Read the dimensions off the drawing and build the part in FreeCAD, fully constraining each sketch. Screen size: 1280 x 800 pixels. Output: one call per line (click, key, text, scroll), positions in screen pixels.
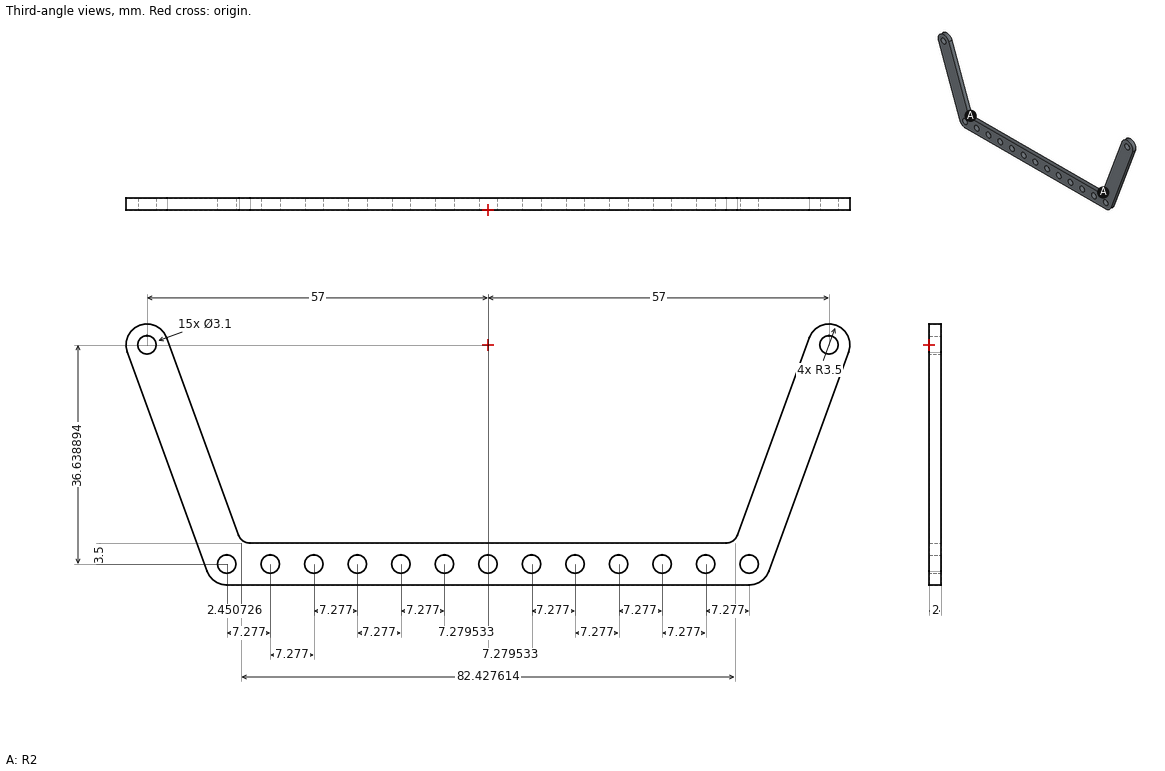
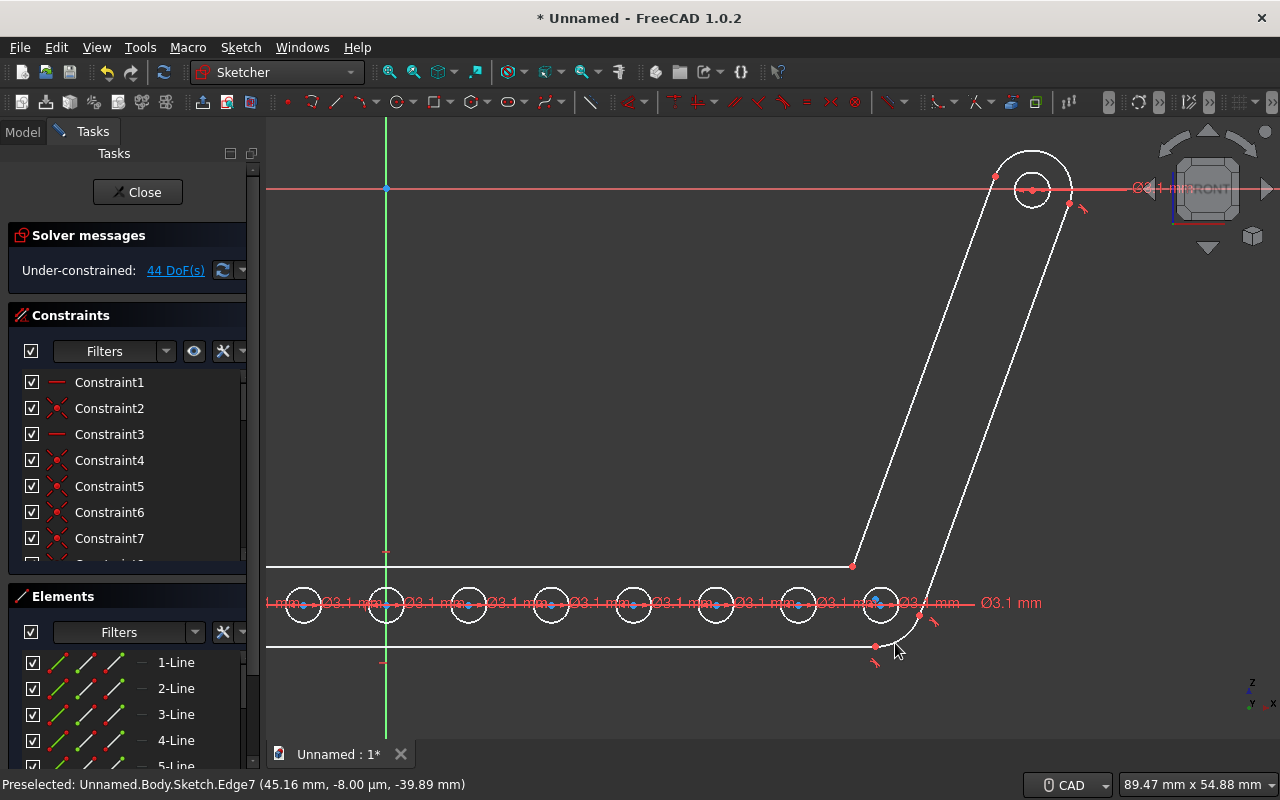
click(580, 647)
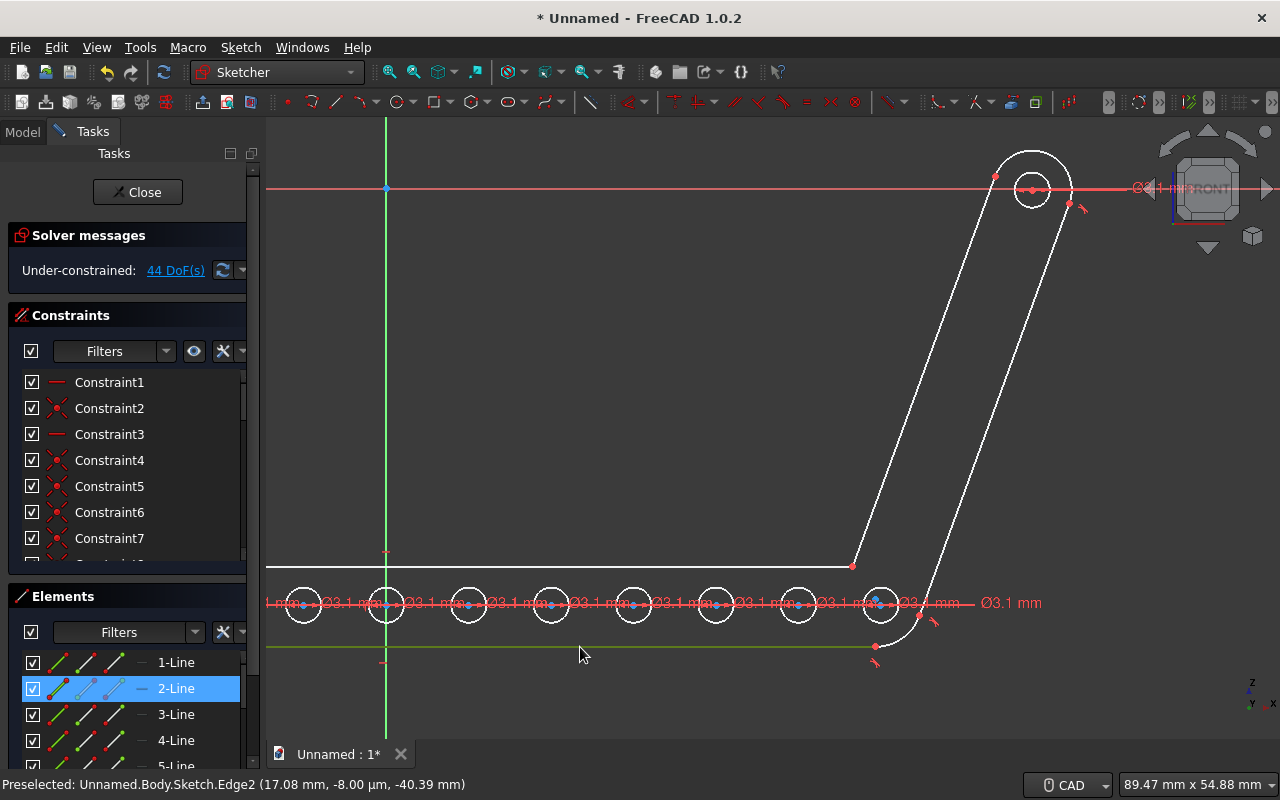
scroll(964, 453, down, 4)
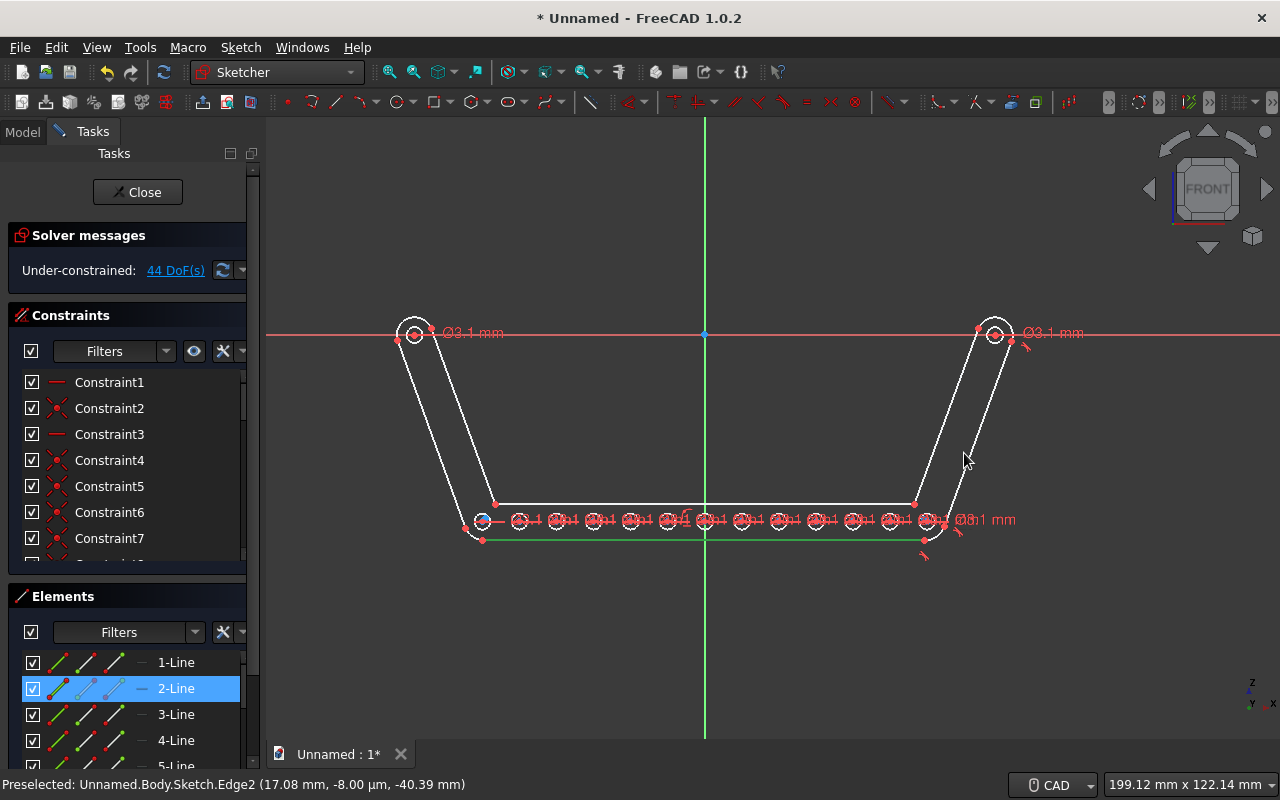
scroll(469, 534, up, 4)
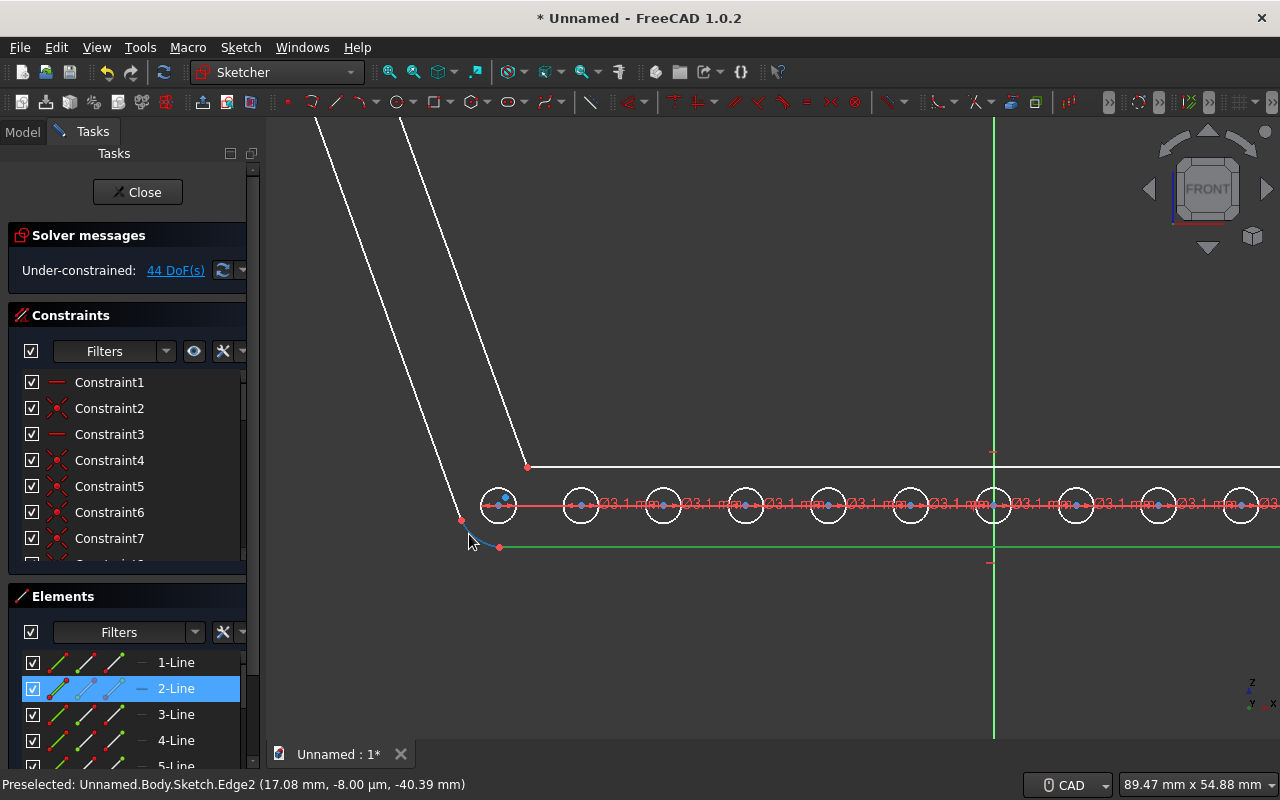
click(470, 532)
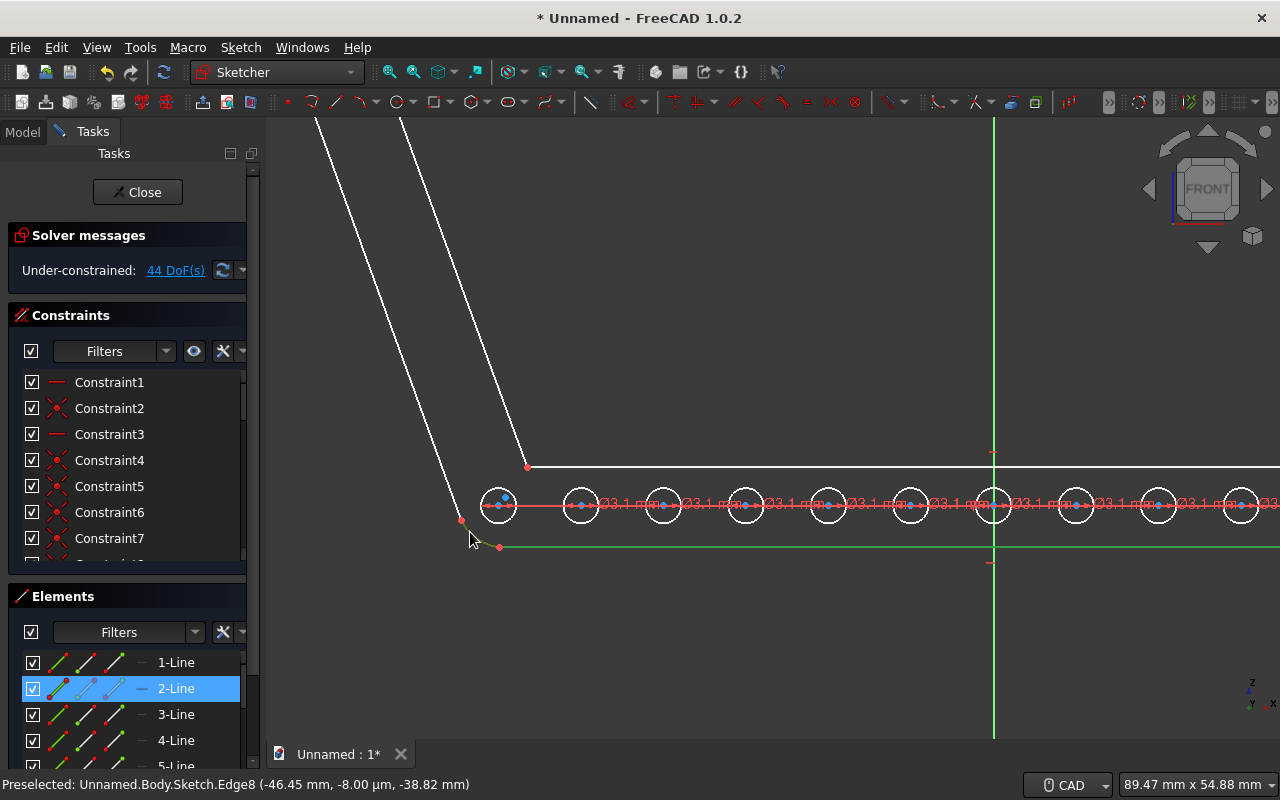
key(t)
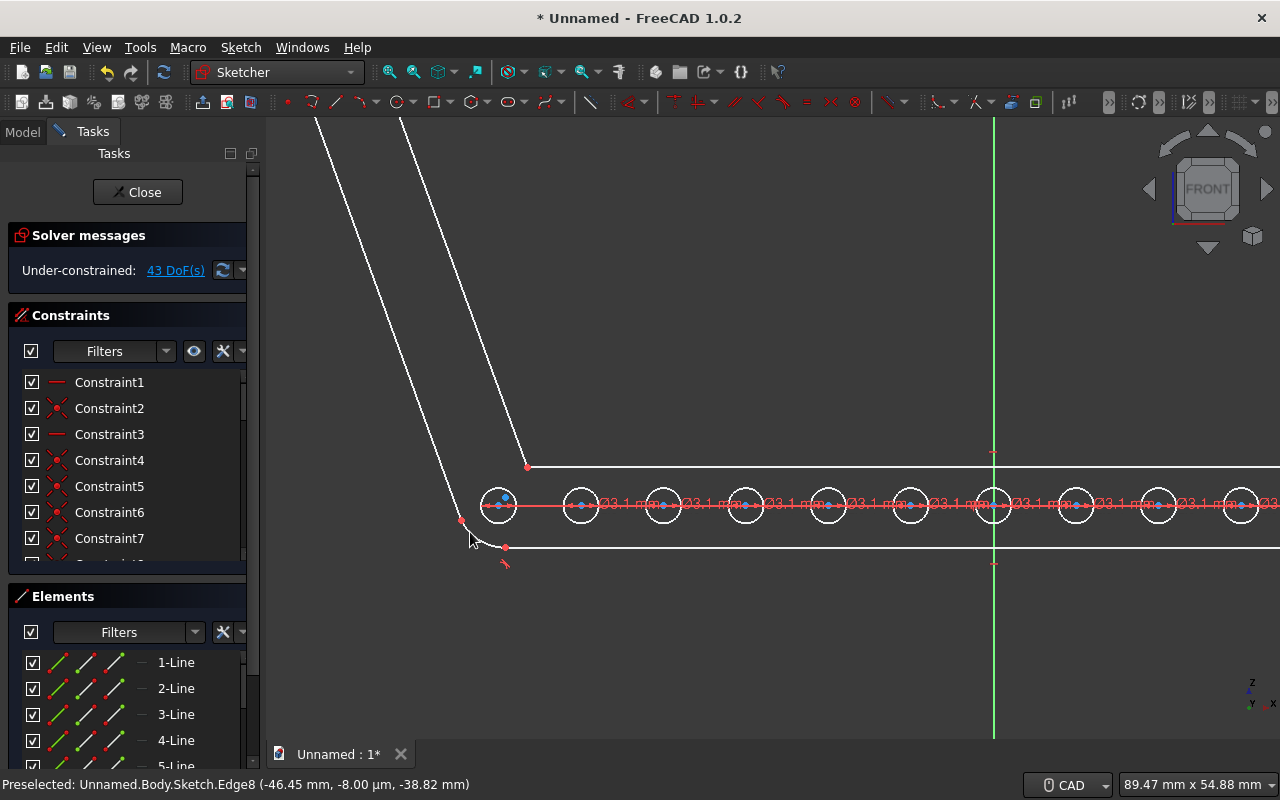
click(416, 396)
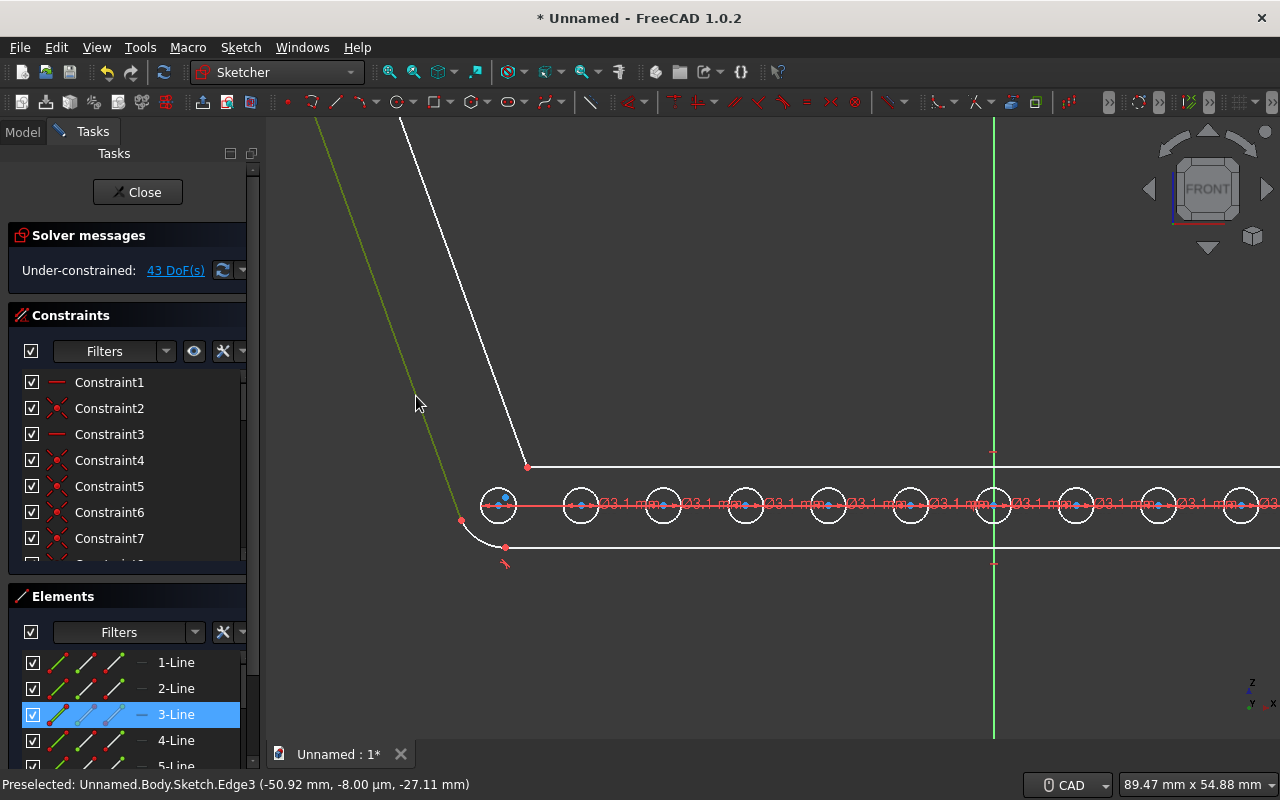
click(471, 534)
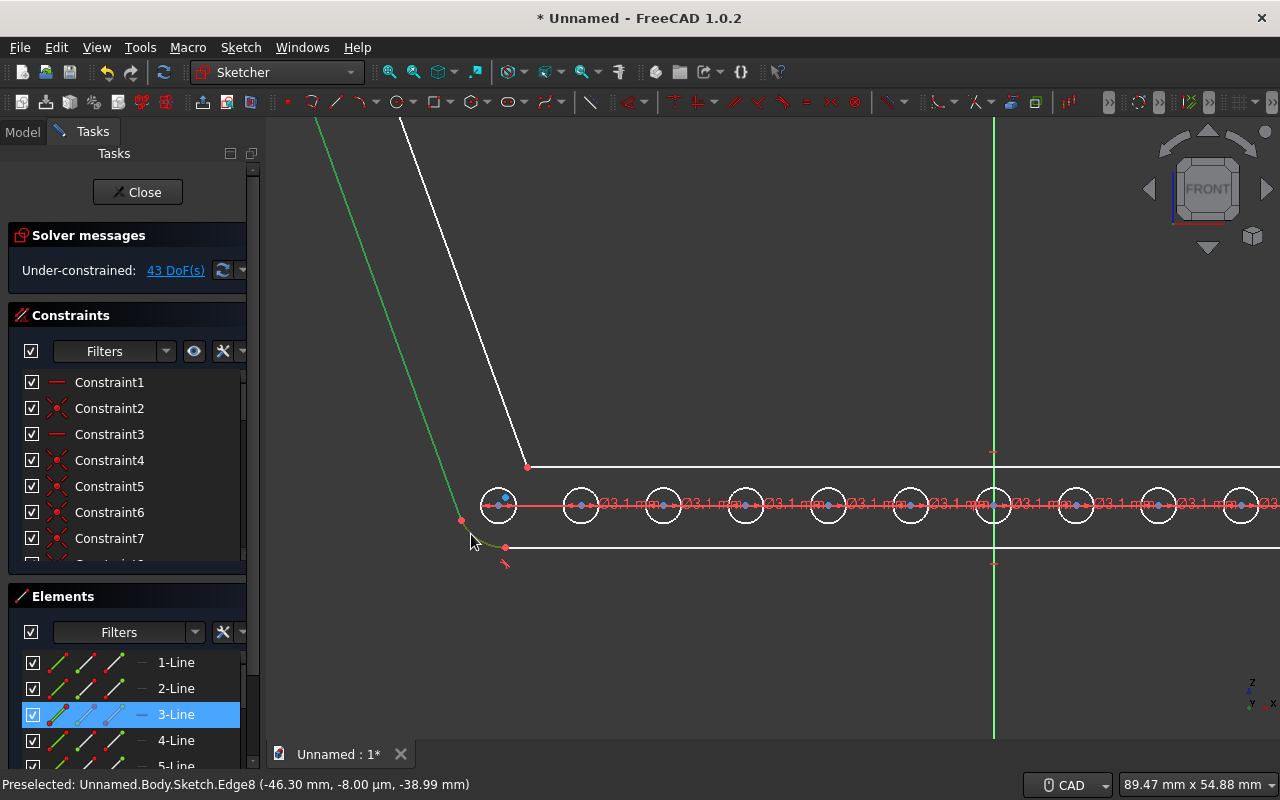
key(t)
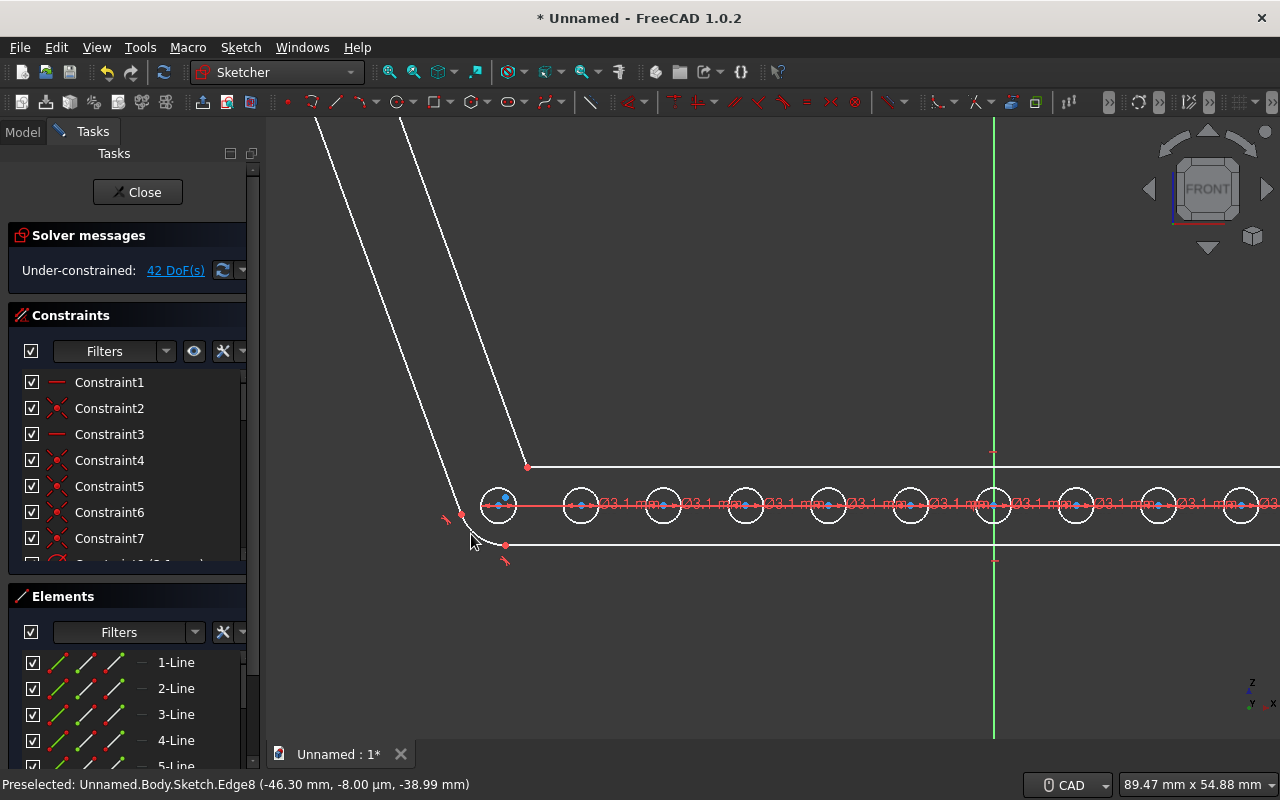
click(416, 391)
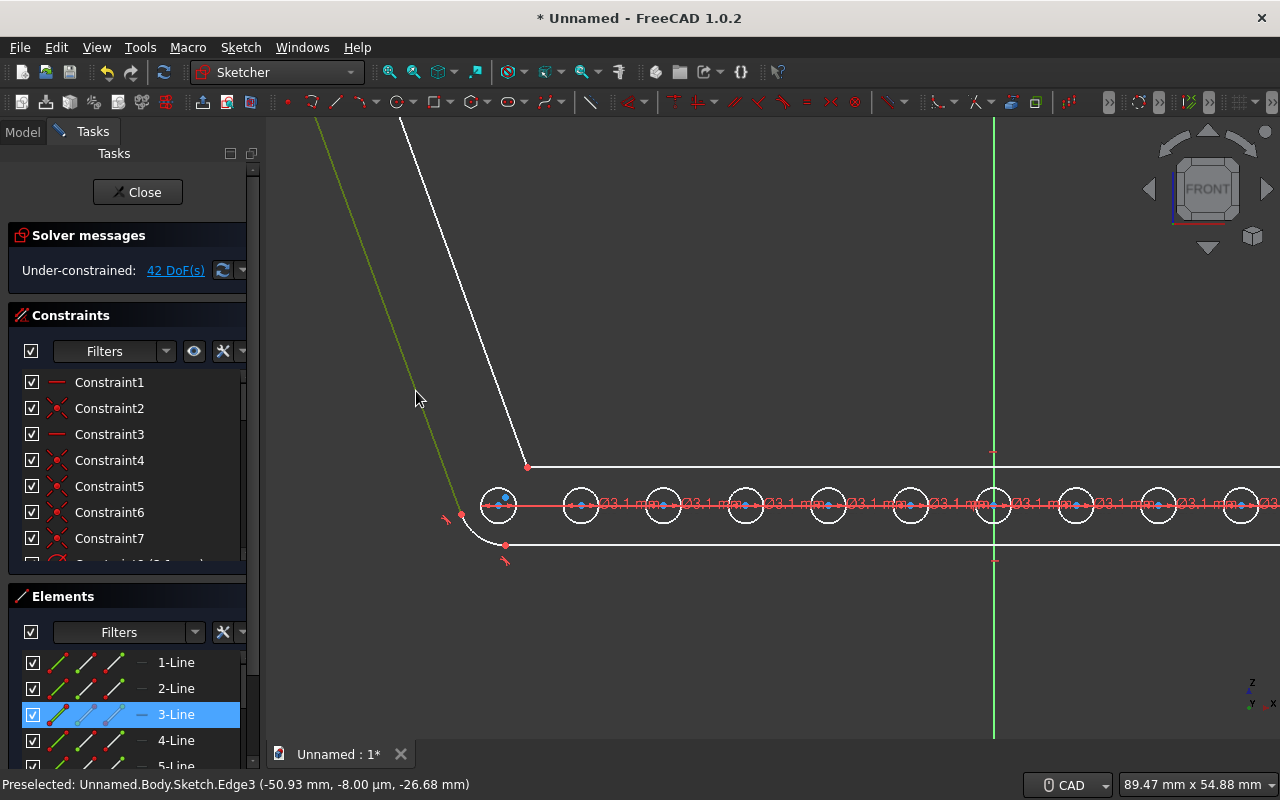
scroll(469, 534, down, 4)